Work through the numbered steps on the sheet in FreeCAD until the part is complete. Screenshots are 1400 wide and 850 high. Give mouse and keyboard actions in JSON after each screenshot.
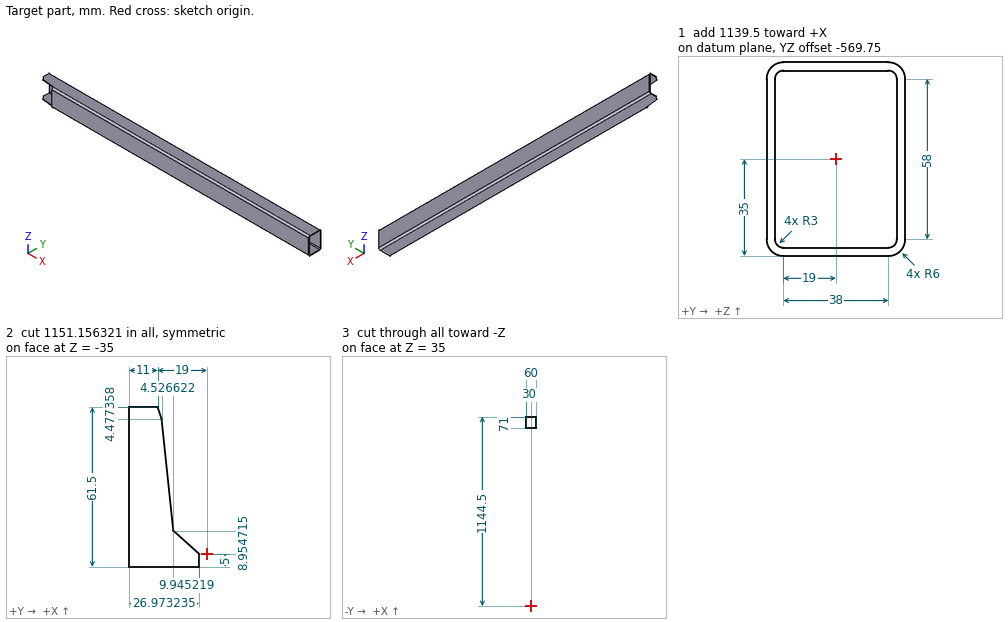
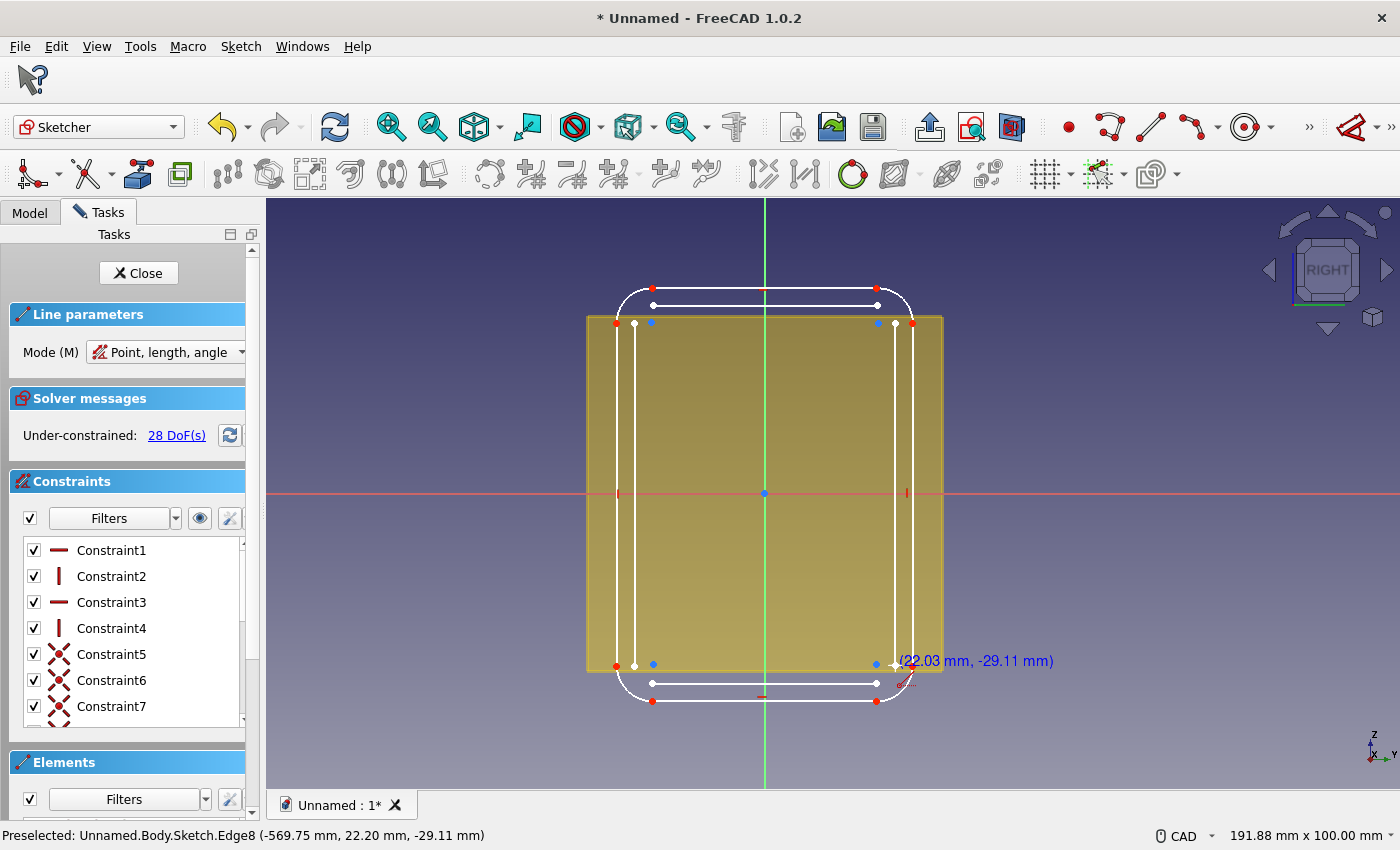
{"action": "key", "text": "g 3 a"}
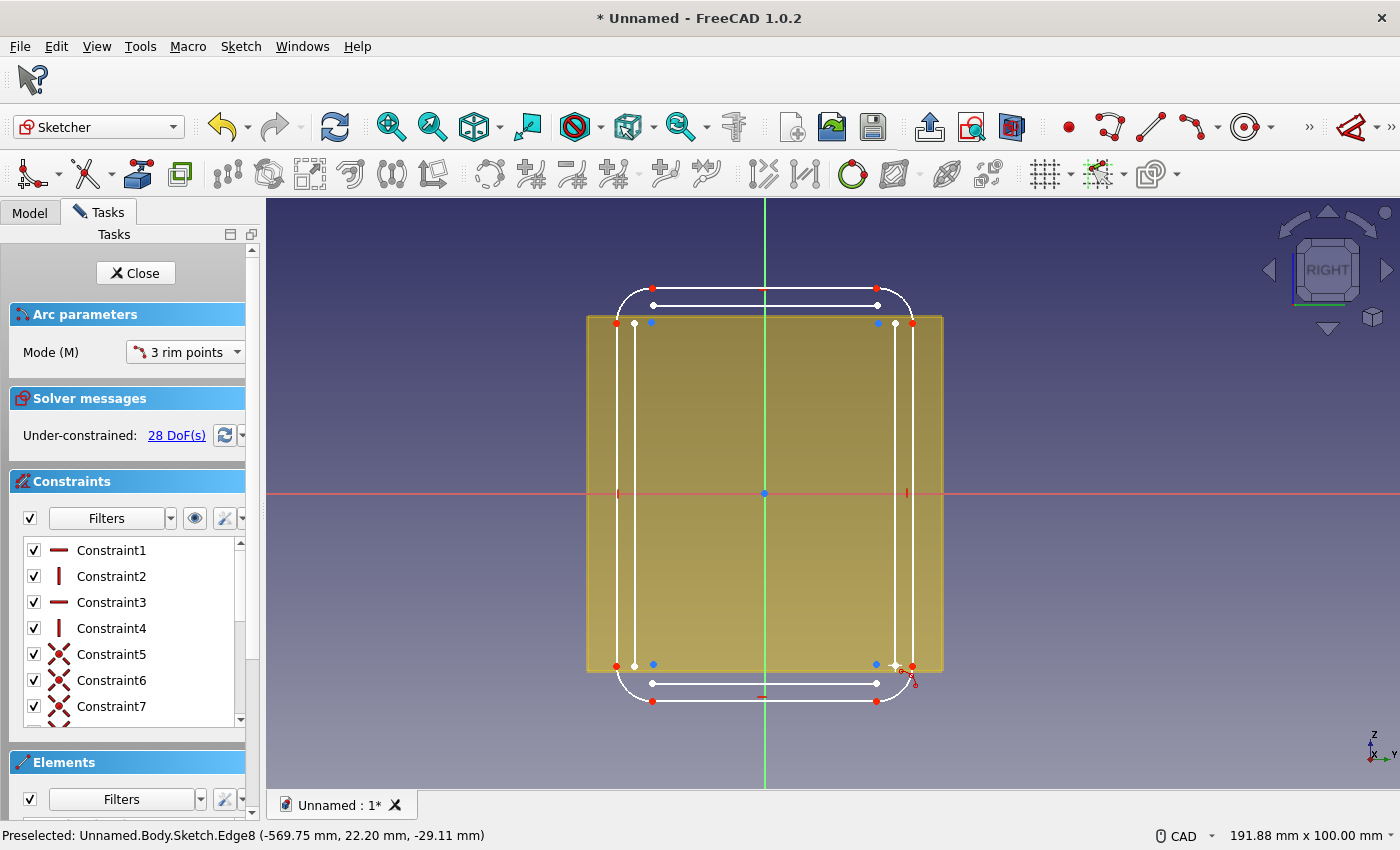
{"action": "left_click", "coordinate": [652, 684]}
{"action": "left_click", "coordinate": [635, 666]}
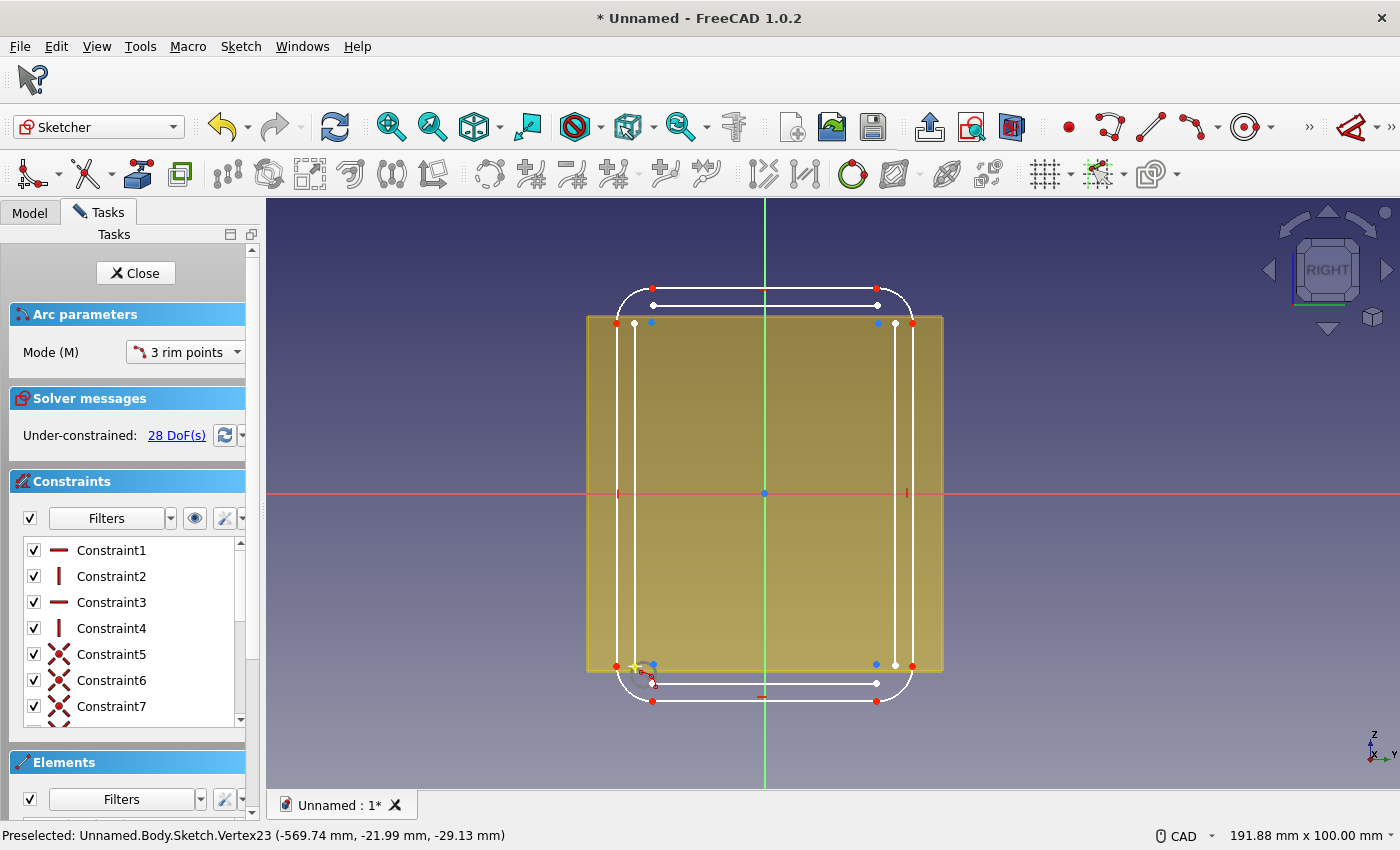
{"action": "scroll", "coordinate": [640, 678], "scroll_direction": "up", "scroll_amount": 6}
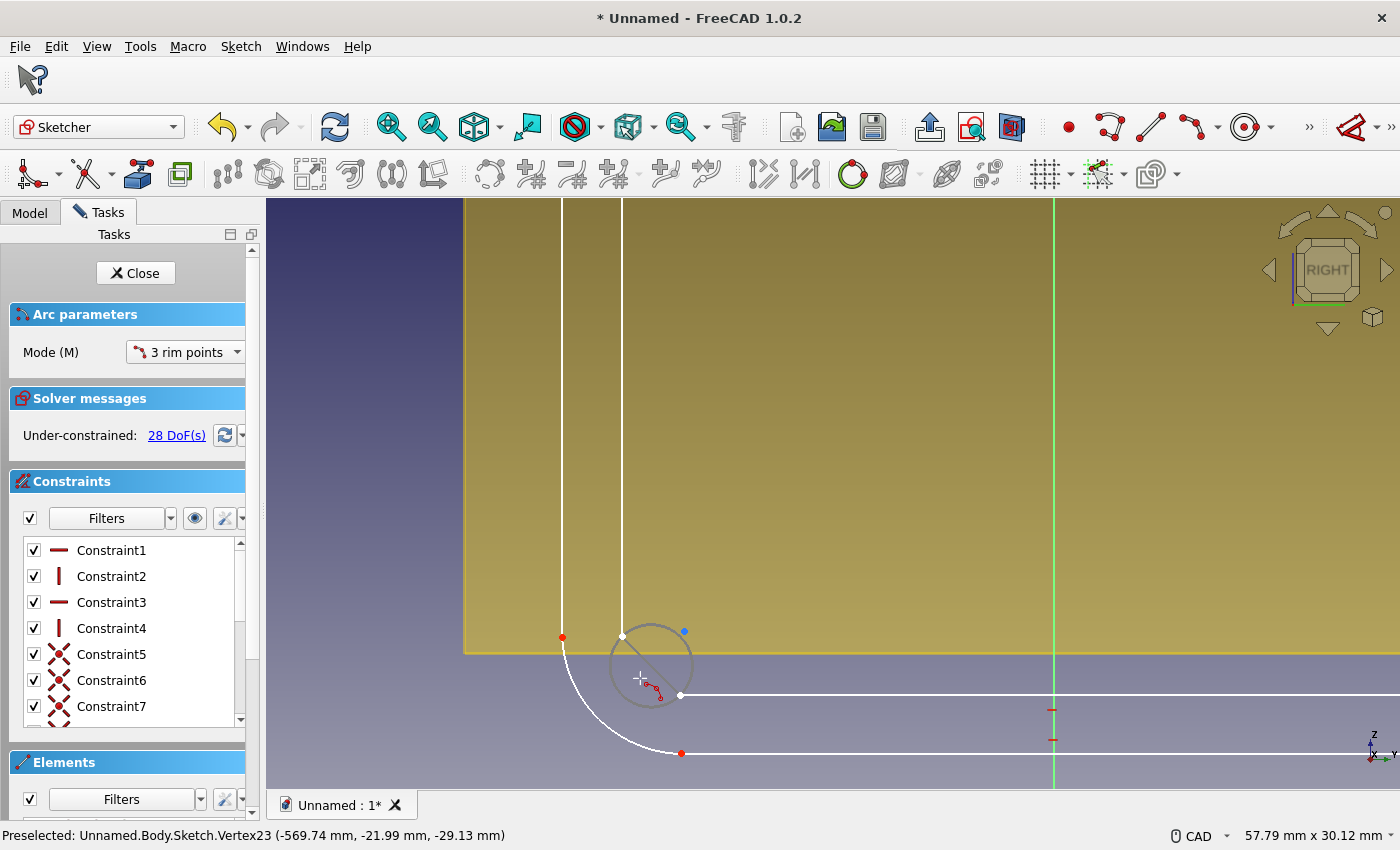
{"action": "left_click", "coordinate": [639, 676]}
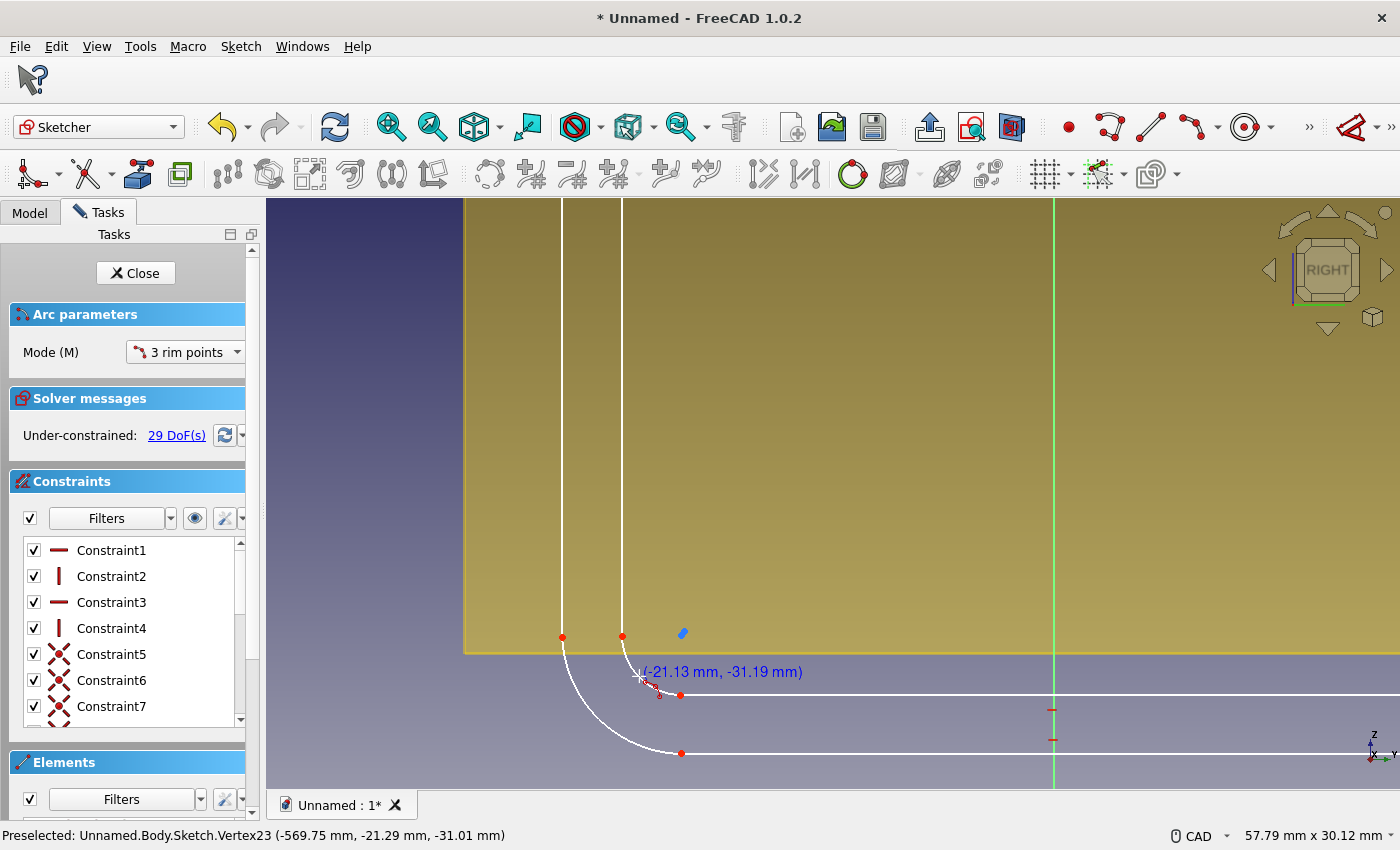
{"action": "scroll", "coordinate": [640, 678], "scroll_direction": "down", "scroll_amount": 6}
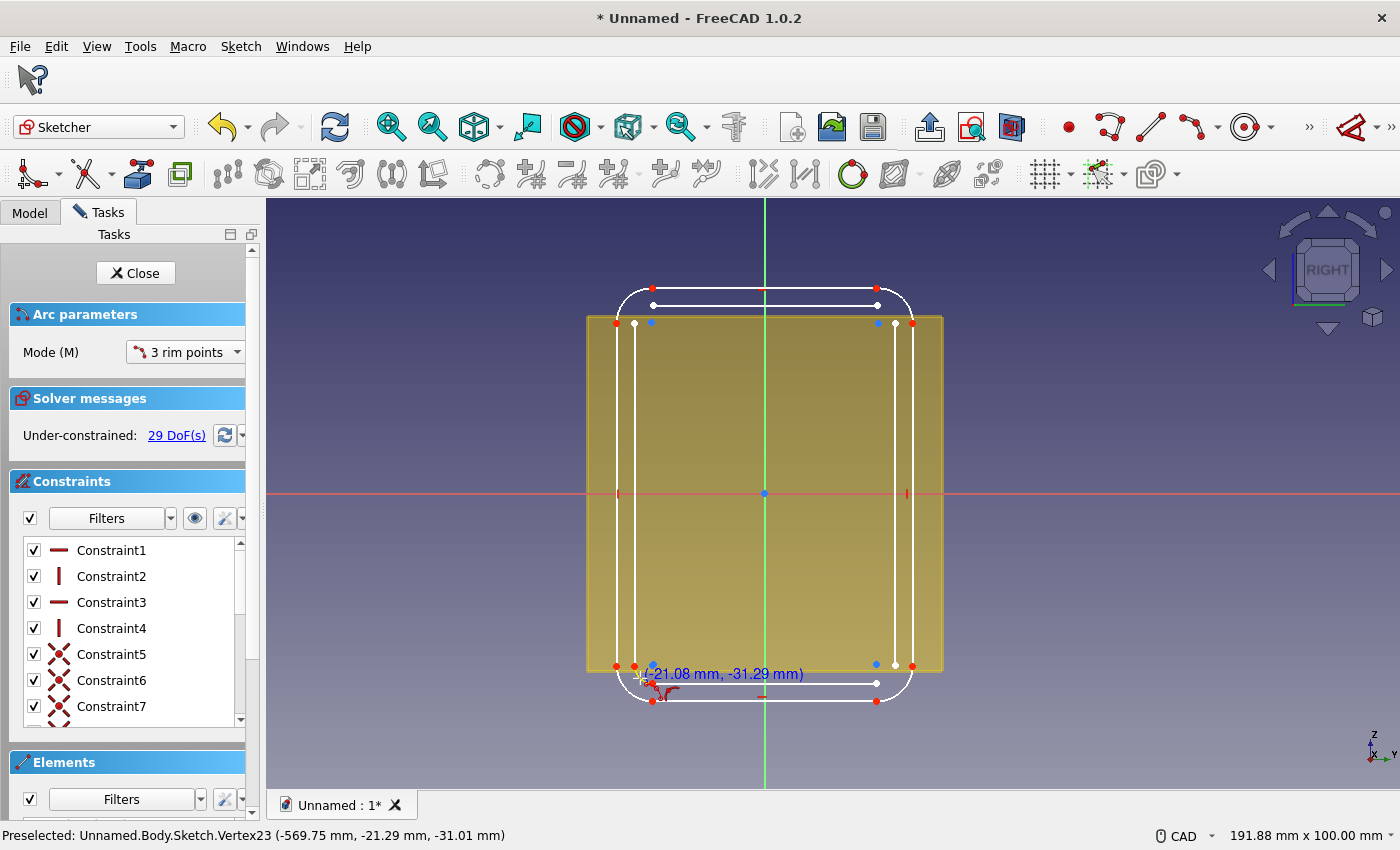
{"action": "left_click", "coordinate": [635, 324]}
{"action": "left_click", "coordinate": [653, 306]}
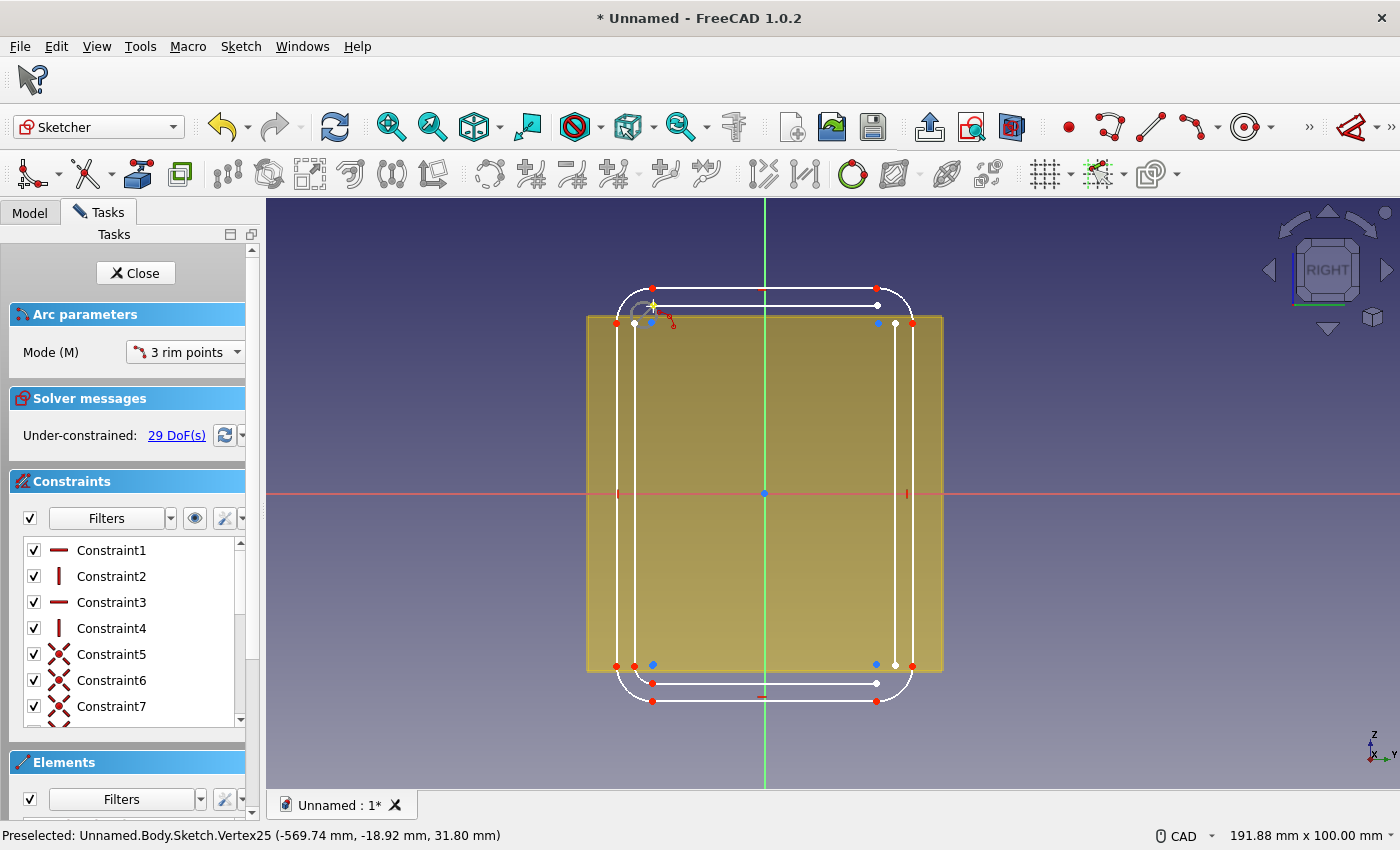
{"action": "scroll", "coordinate": [640, 310], "scroll_direction": "up", "scroll_amount": 6}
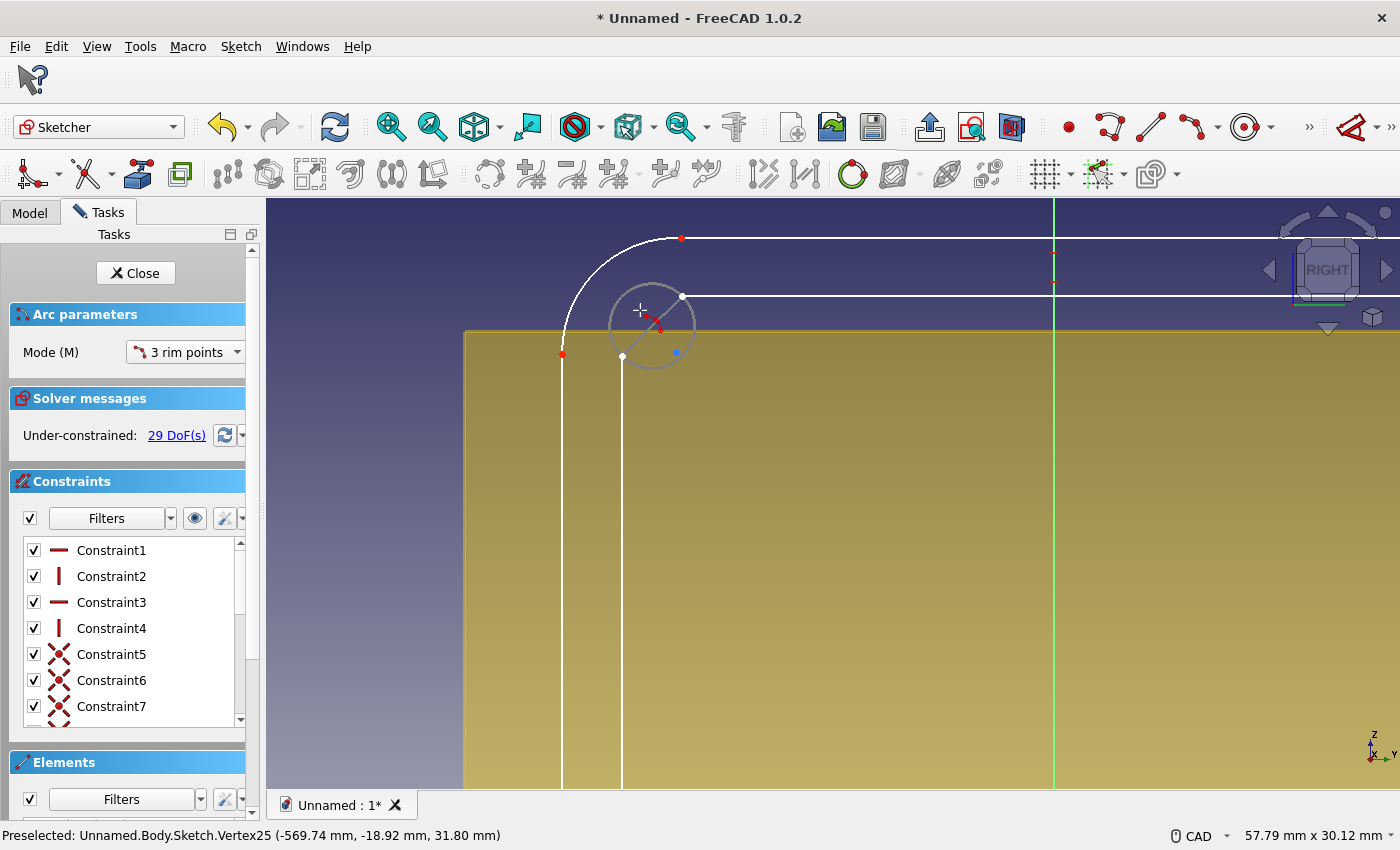
{"action": "left_click", "coordinate": [639, 310]}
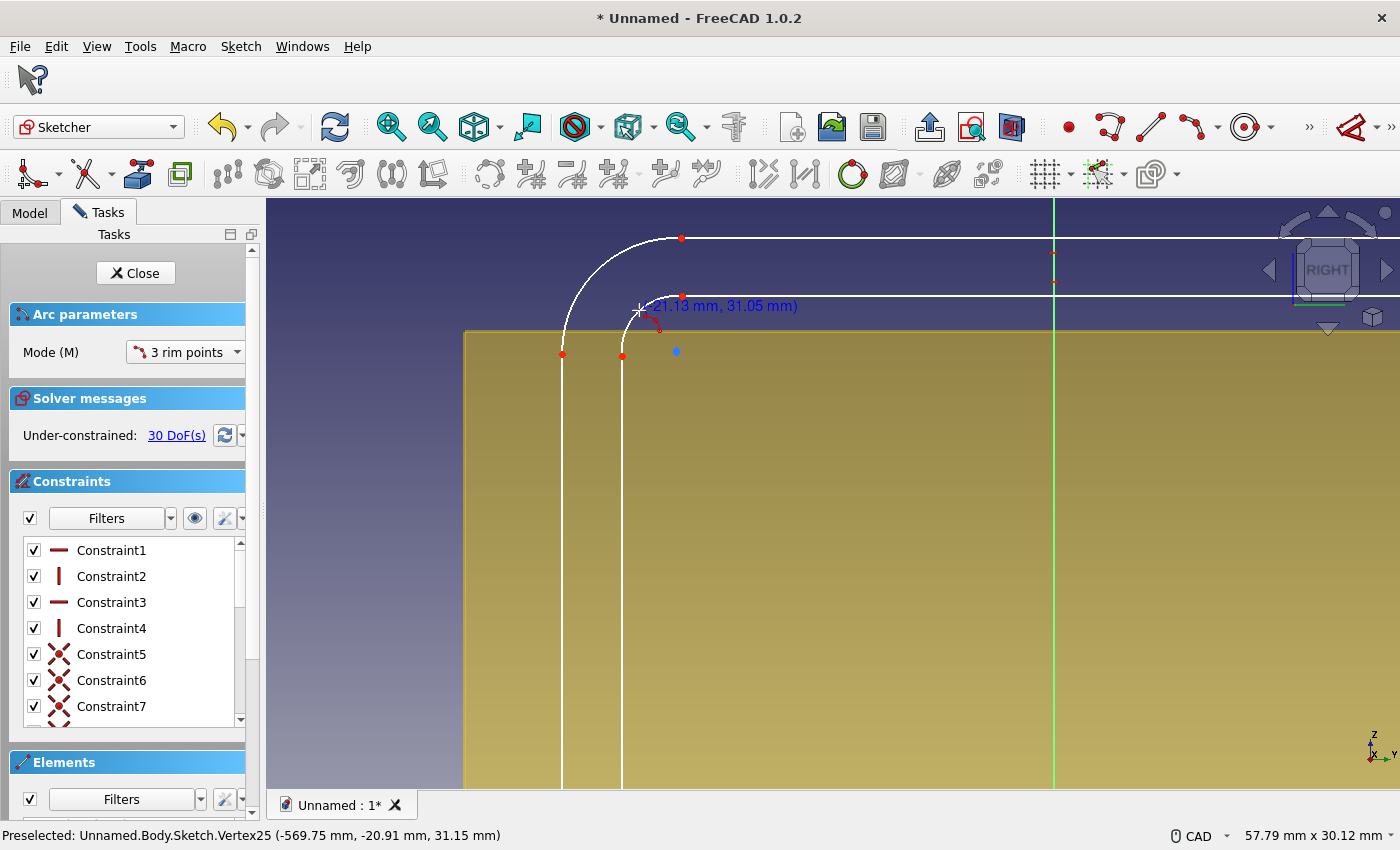
{"action": "scroll", "coordinate": [640, 310], "scroll_direction": "down", "scroll_amount": 6}